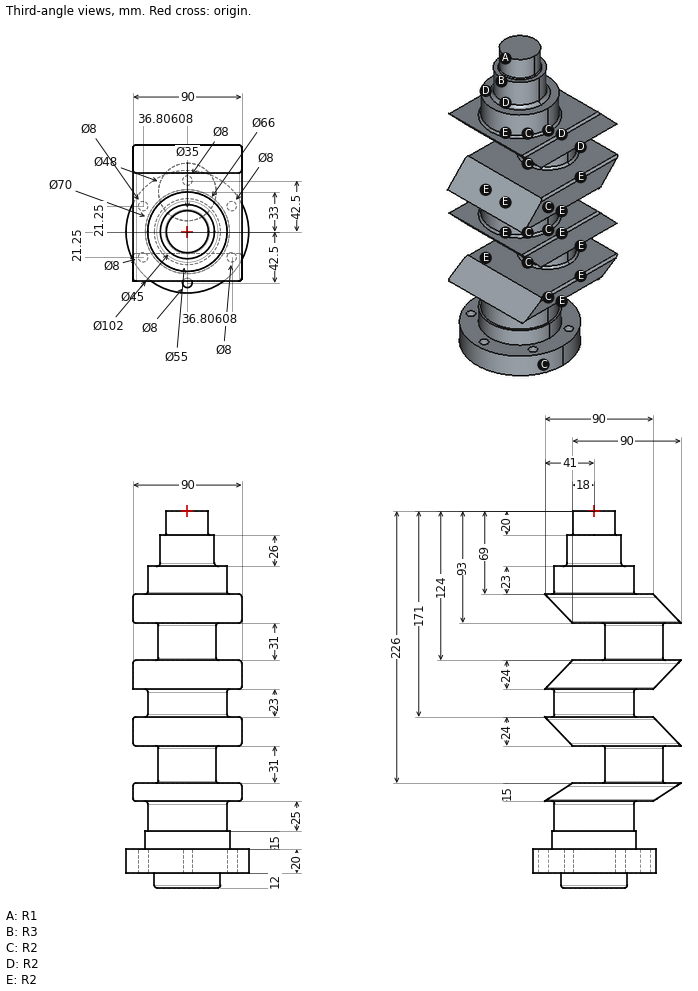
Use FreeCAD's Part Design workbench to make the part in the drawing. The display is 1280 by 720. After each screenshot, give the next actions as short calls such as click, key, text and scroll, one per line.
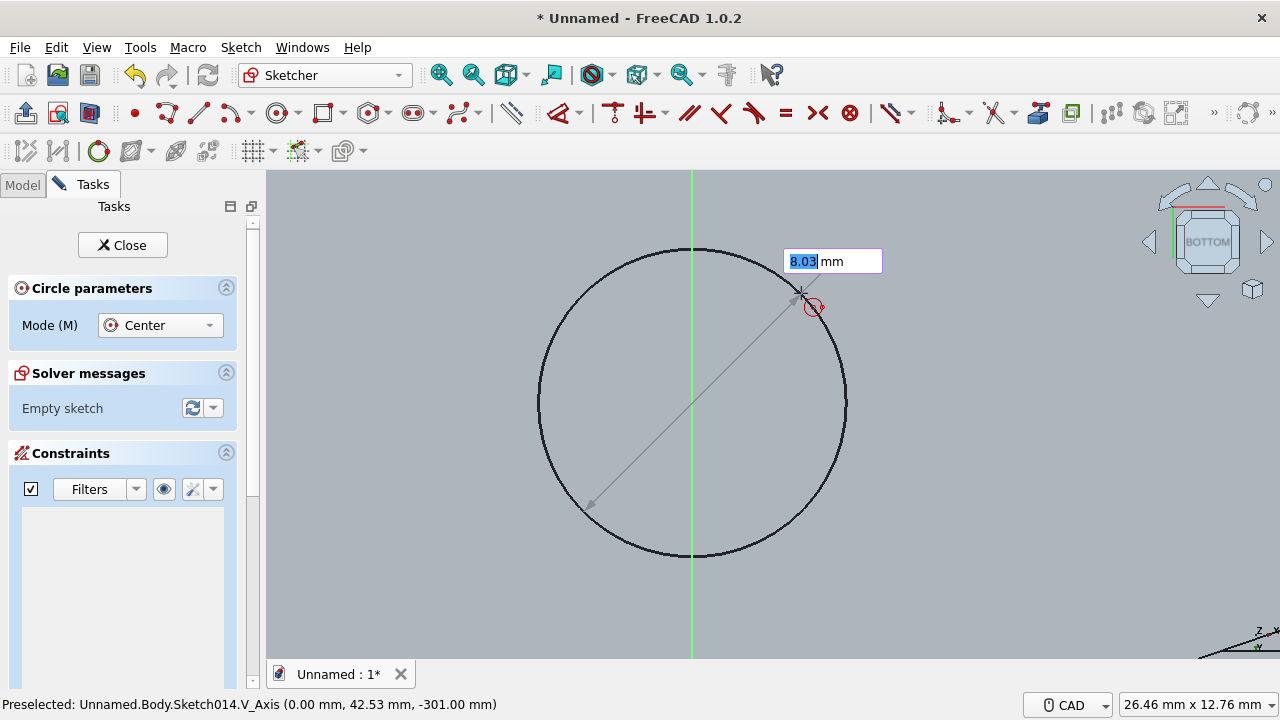
text(8)
key(Return)
key(Escape)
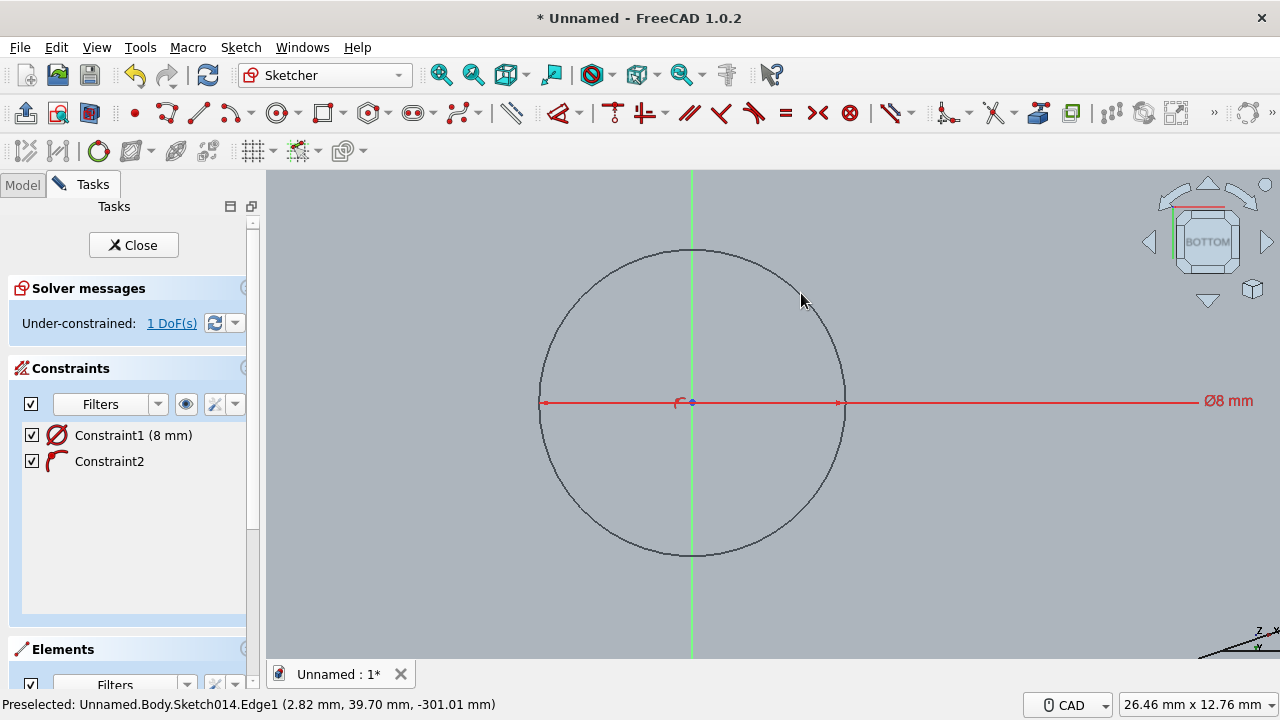
click(558, 114)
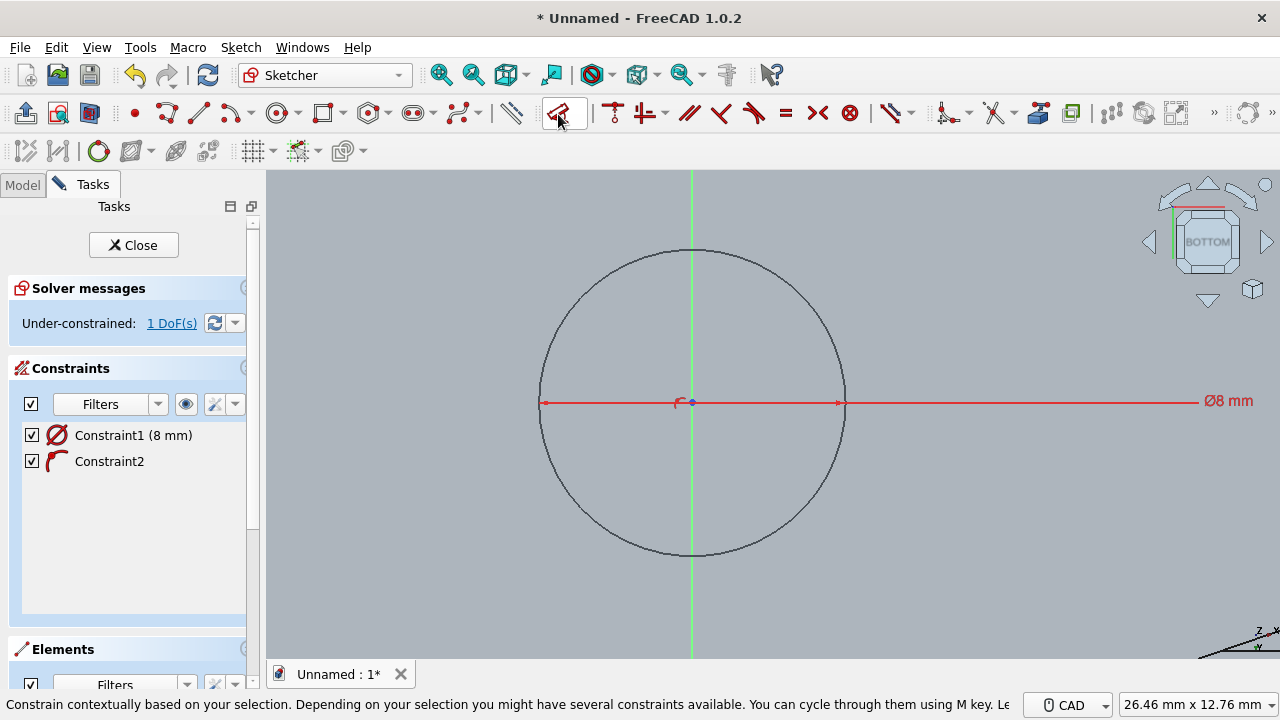
click(692, 403)
click(726, 300)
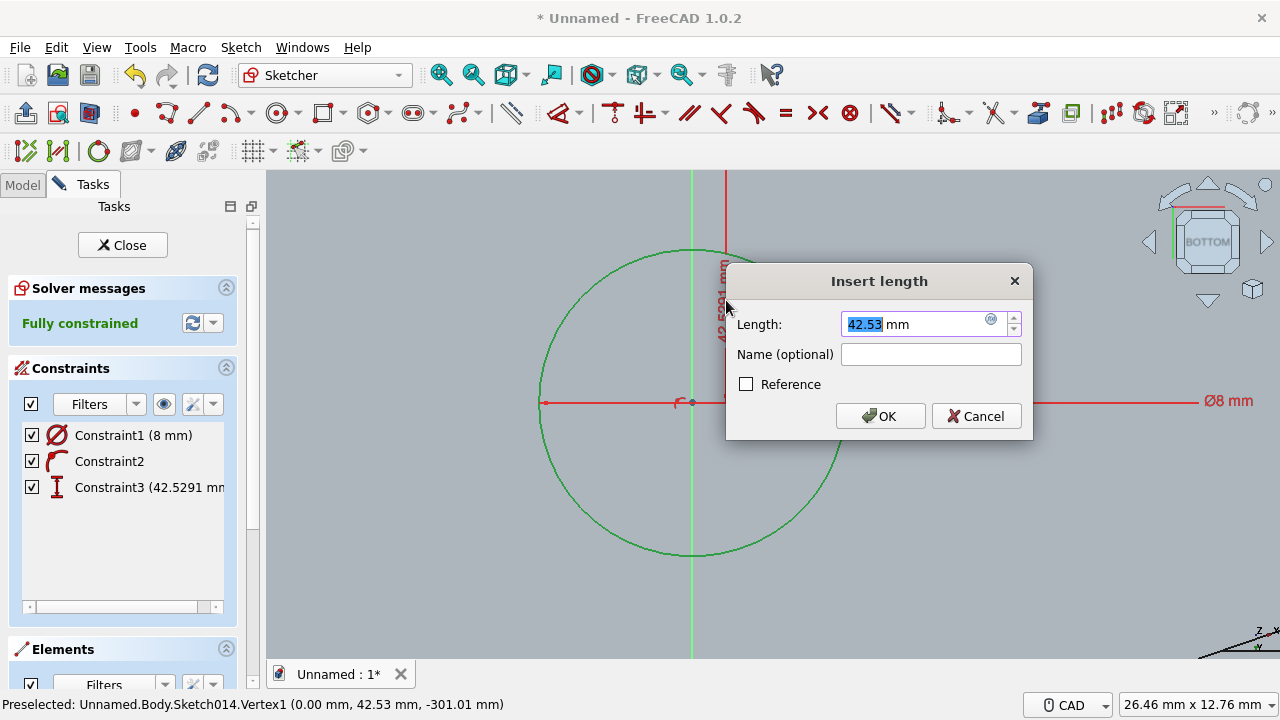
text(42.5)
key(Return)
key(Escape)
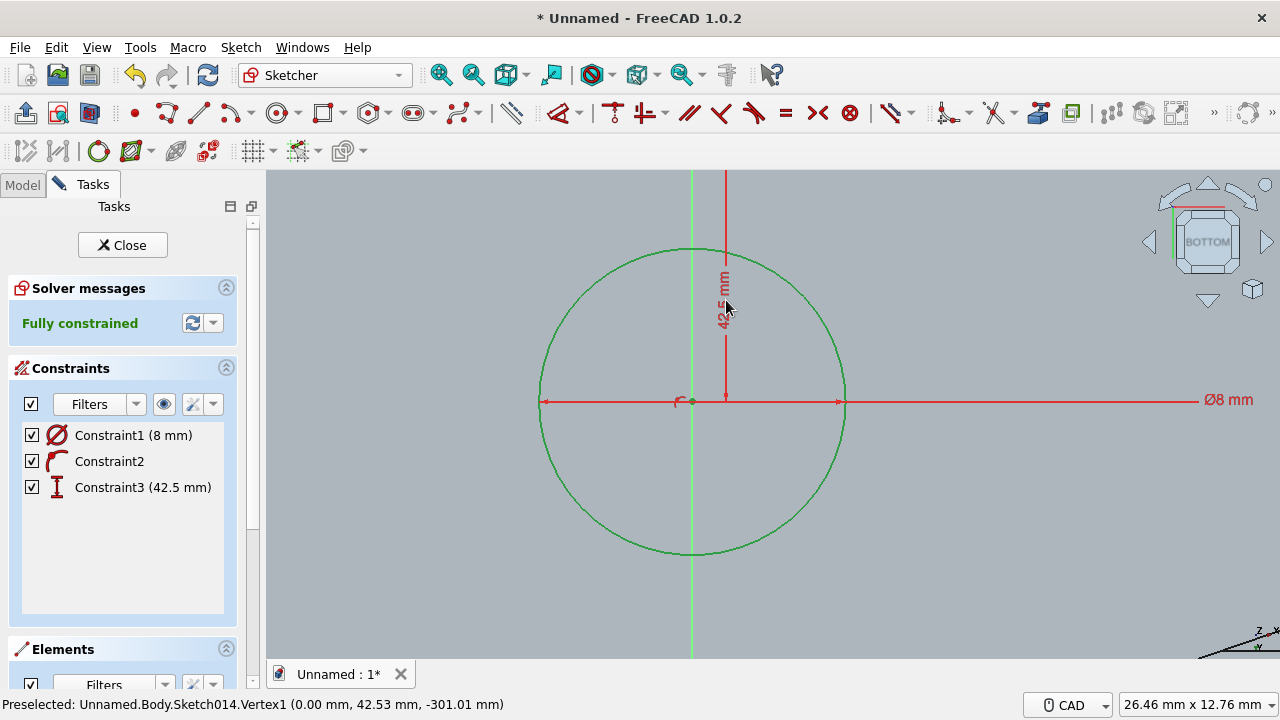
click(123, 245)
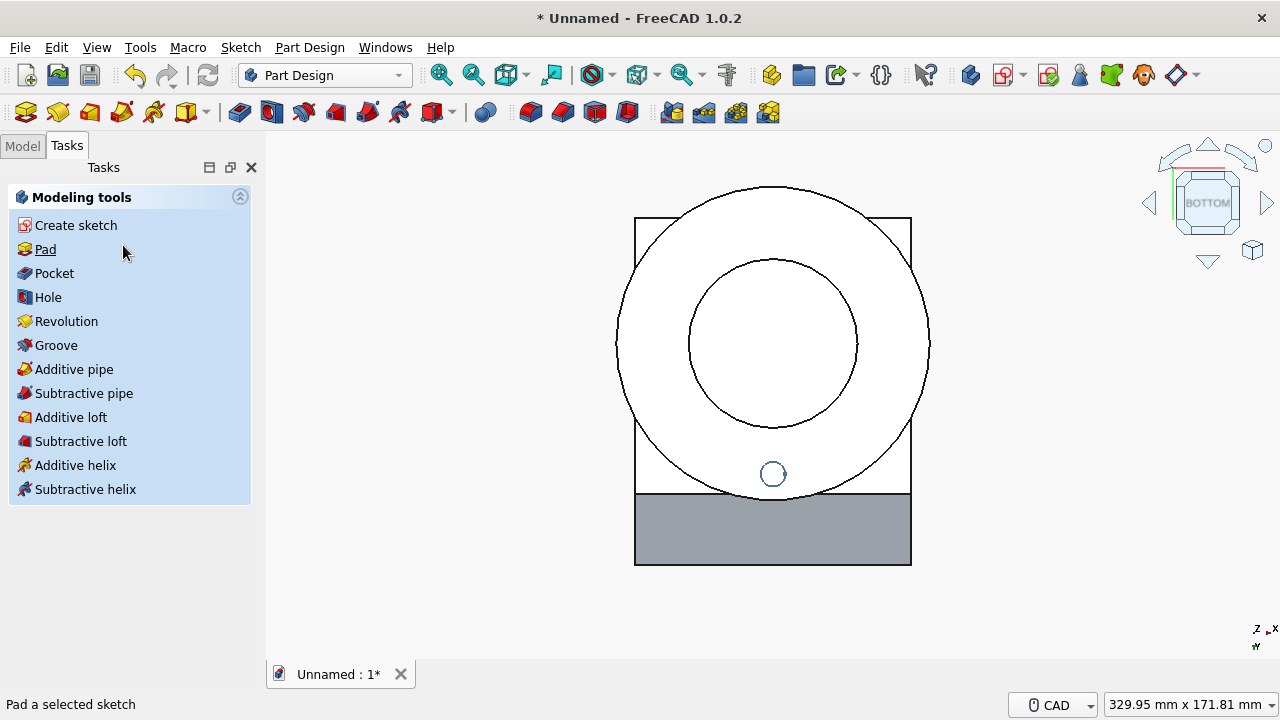
click(240, 112)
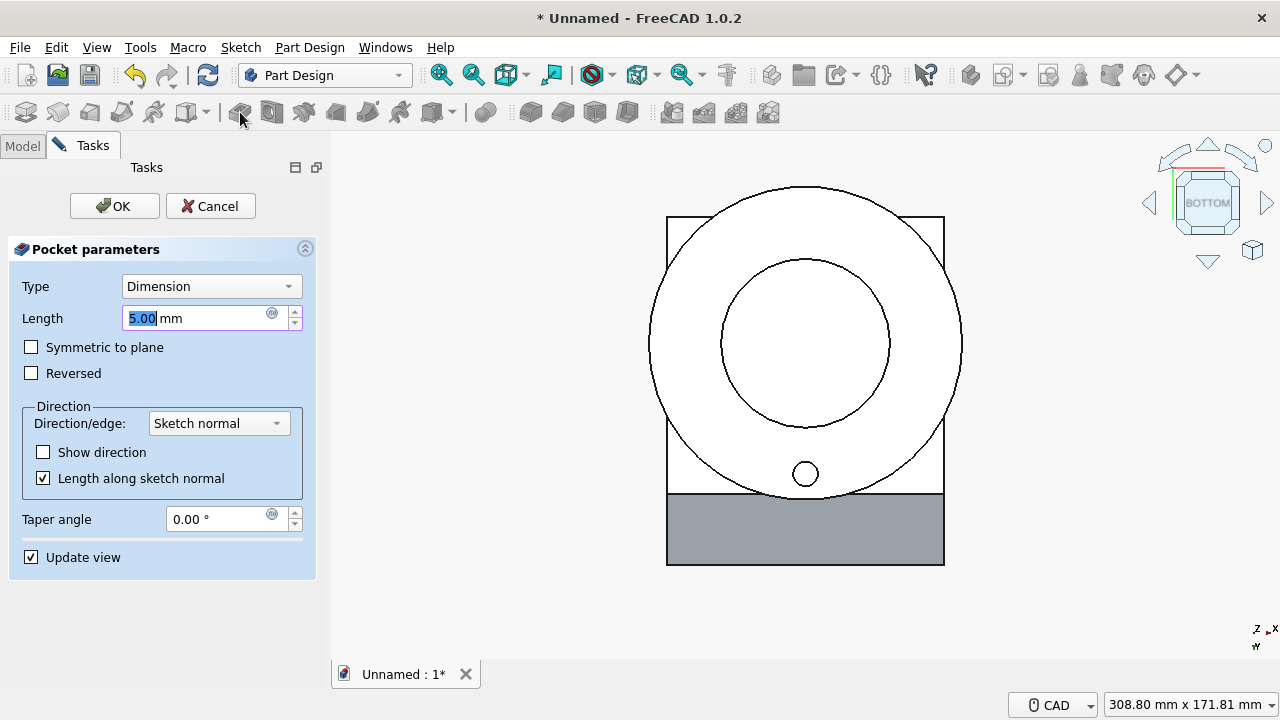
click(212, 286)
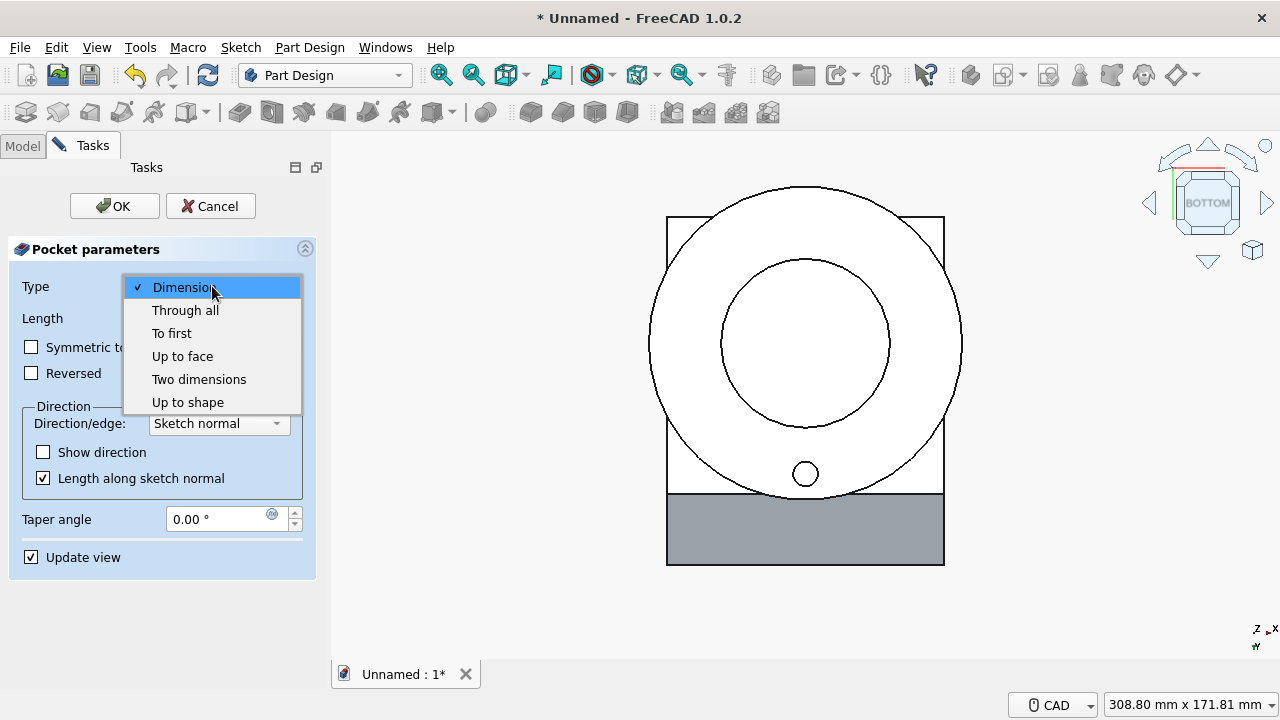
click(212, 334)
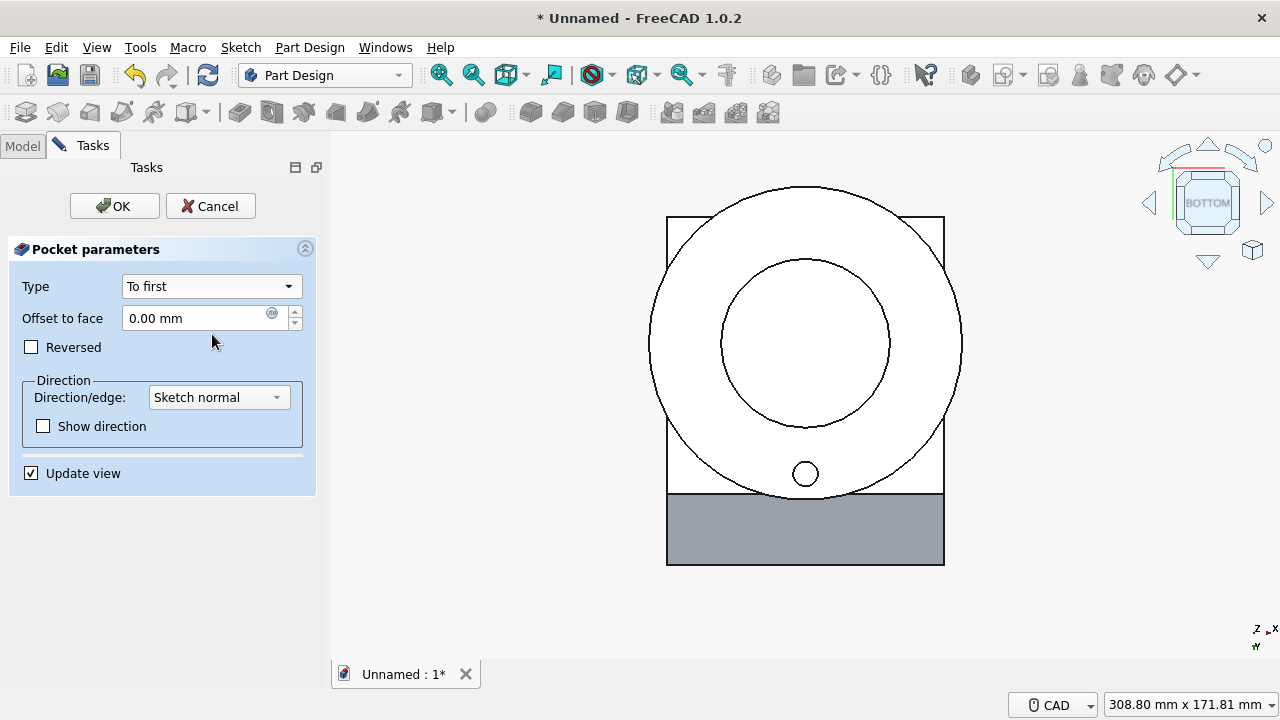
click(115, 206)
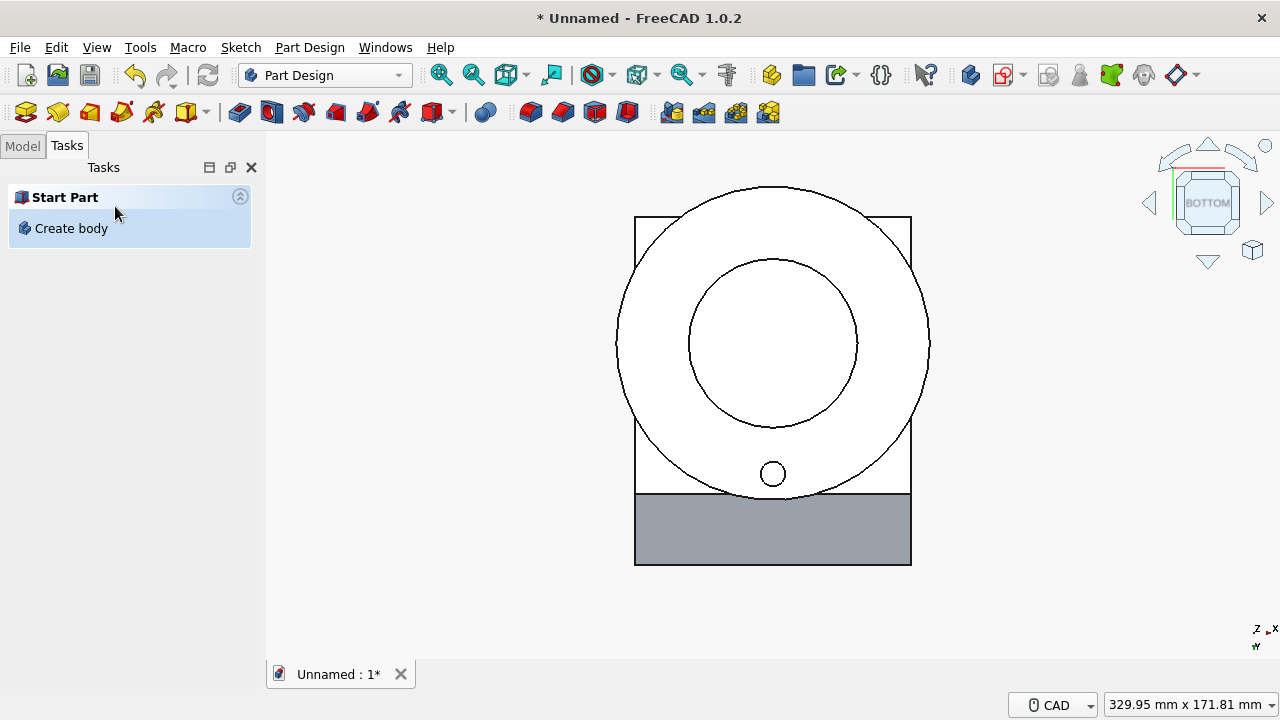
click(863, 432)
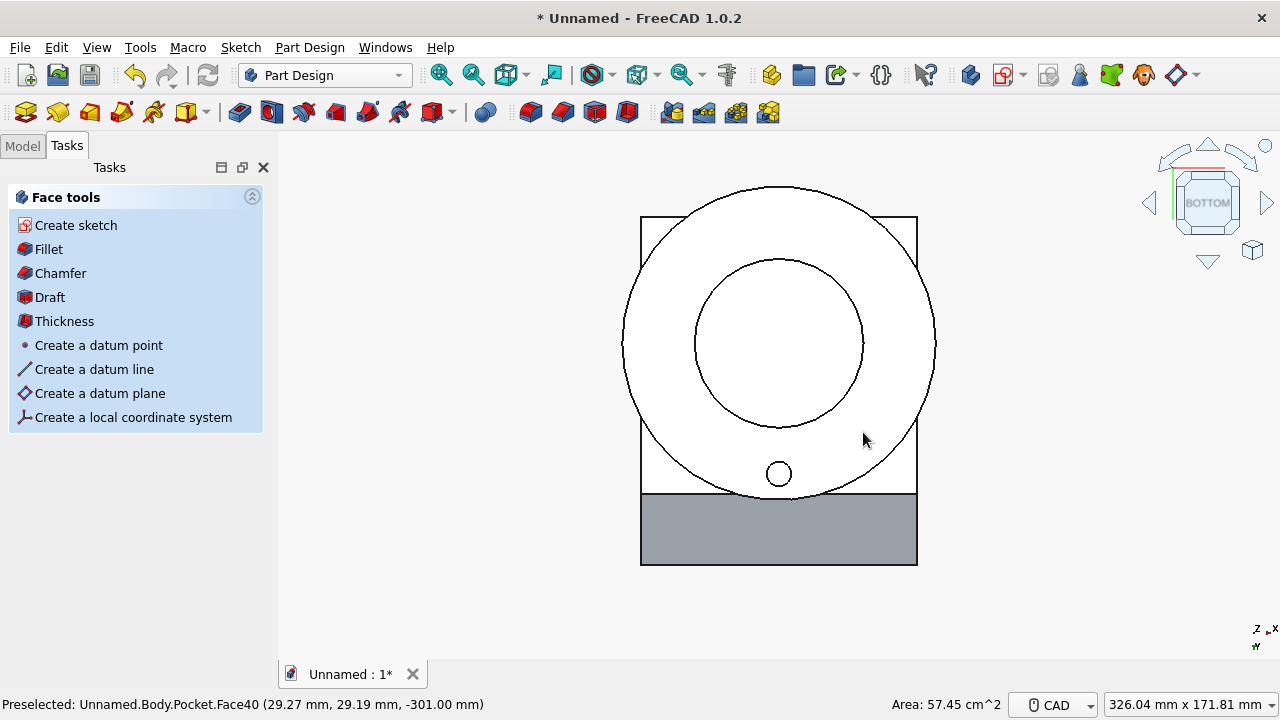
click(1004, 76)